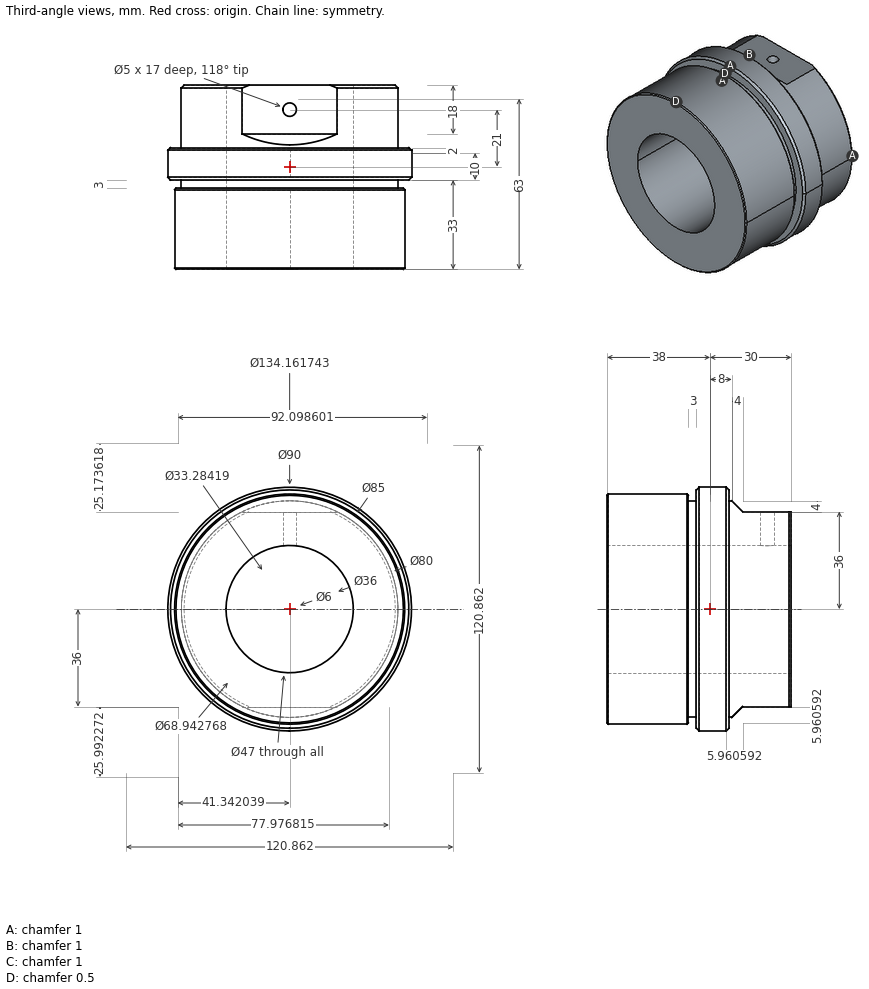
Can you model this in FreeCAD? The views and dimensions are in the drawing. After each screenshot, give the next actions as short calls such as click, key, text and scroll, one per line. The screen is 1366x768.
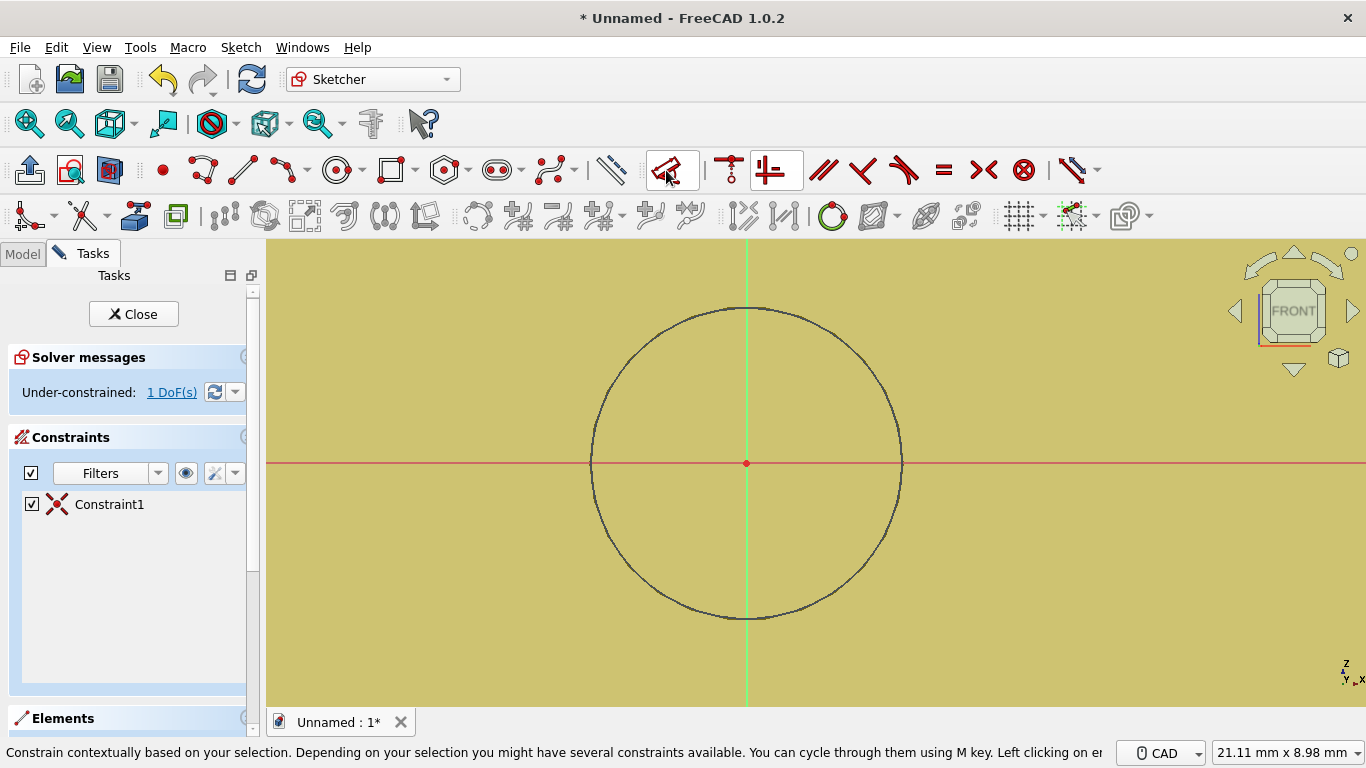
click(856, 353)
click(879, 330)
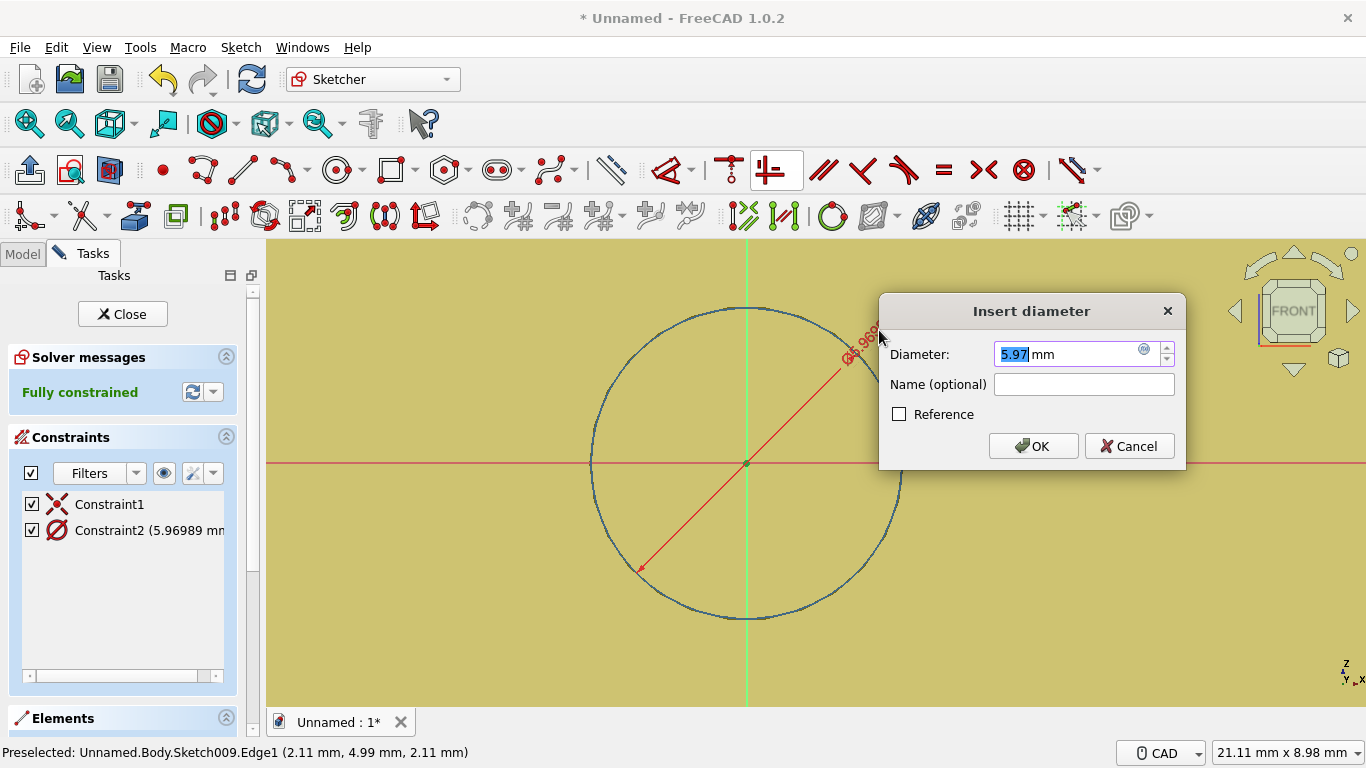
text(6)
key(Return)
key(Escape)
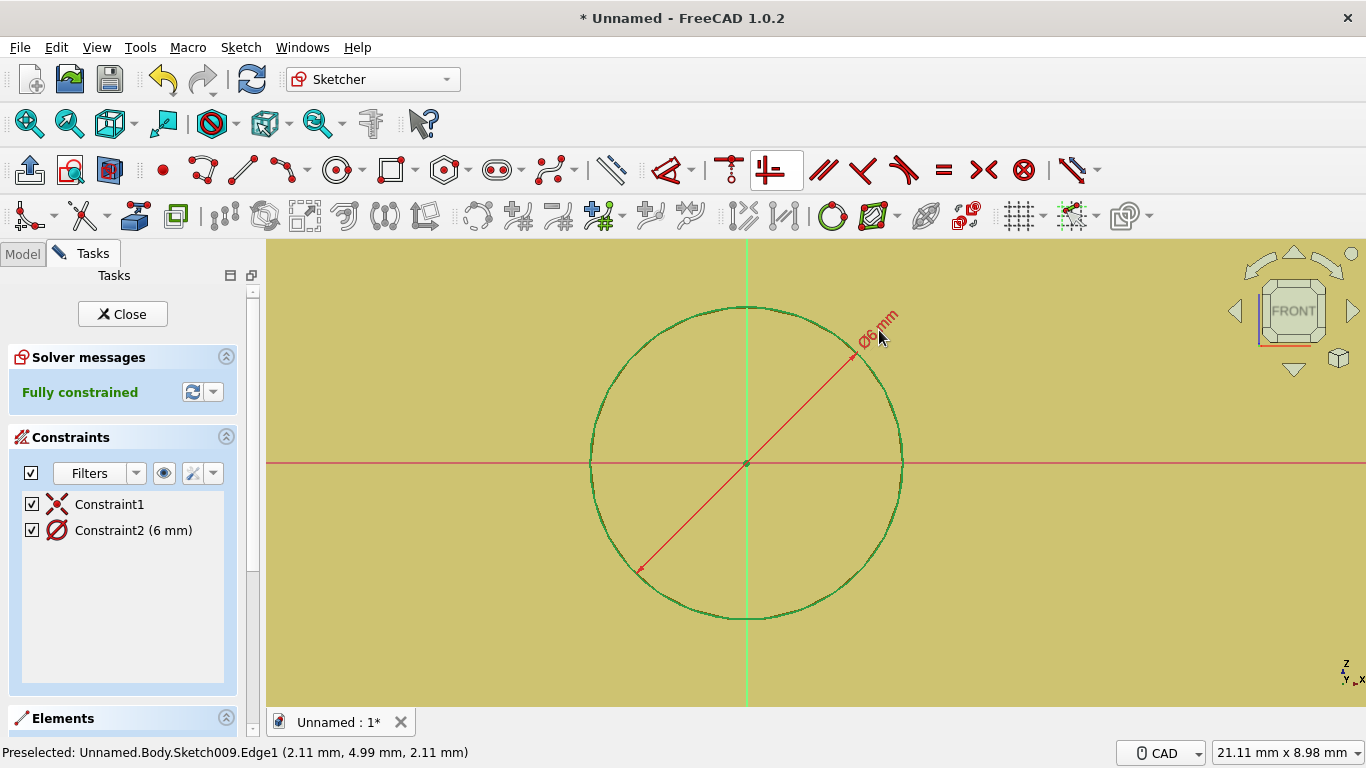
click(123, 314)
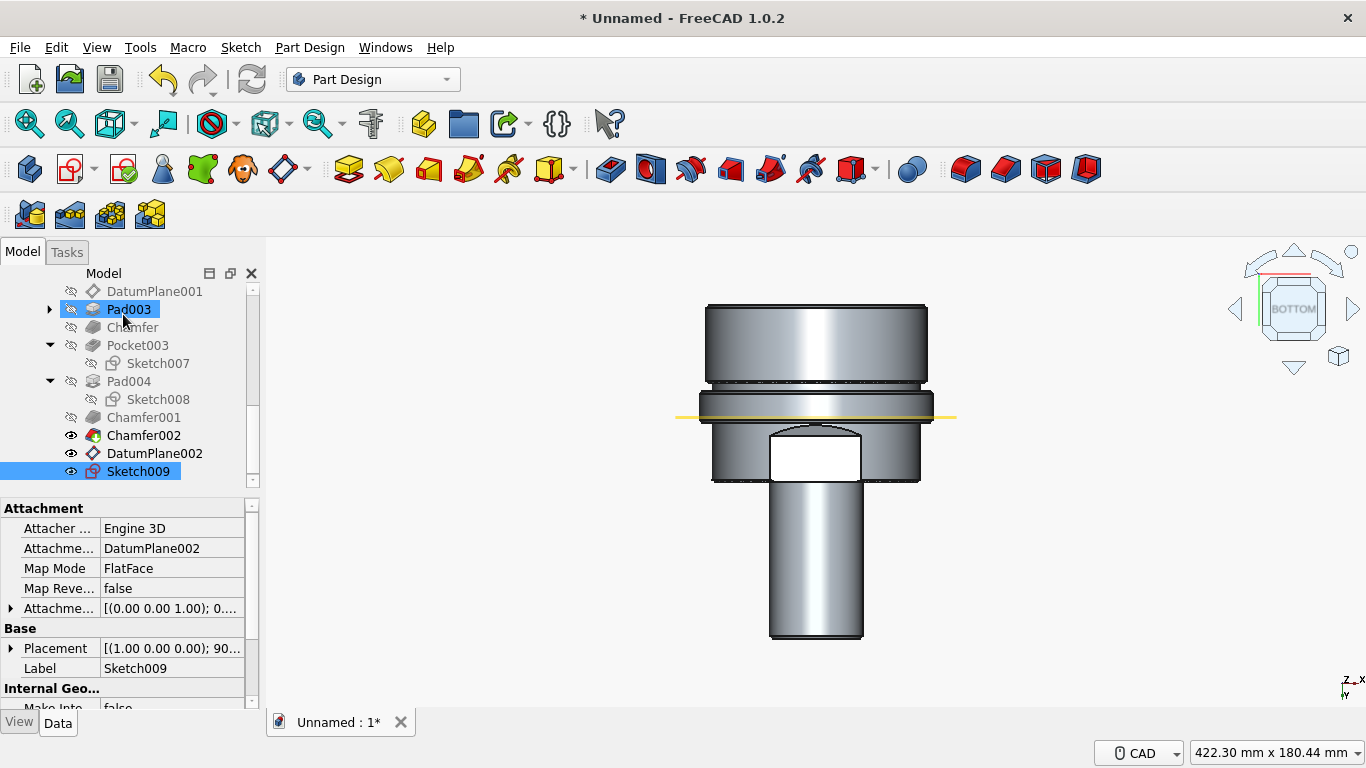
click(612, 170)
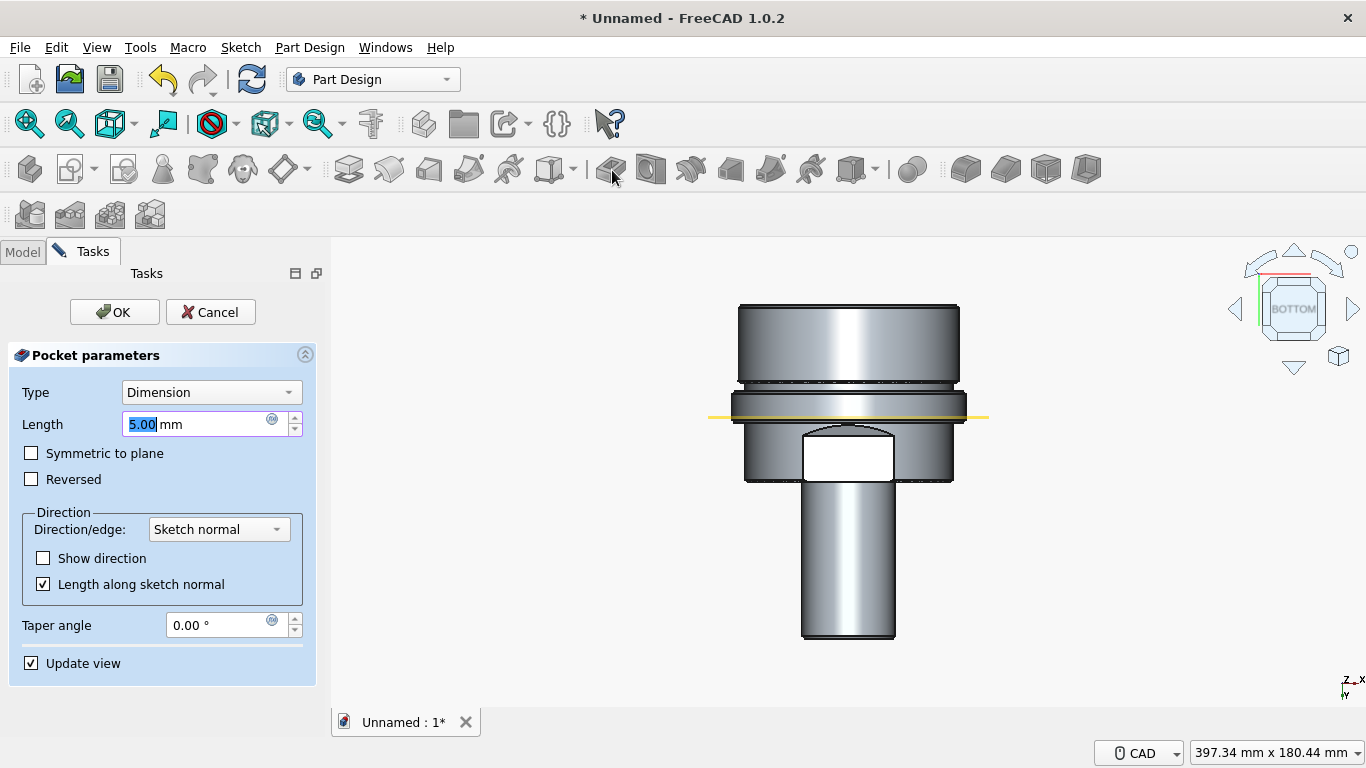
text(2)
key(Tab)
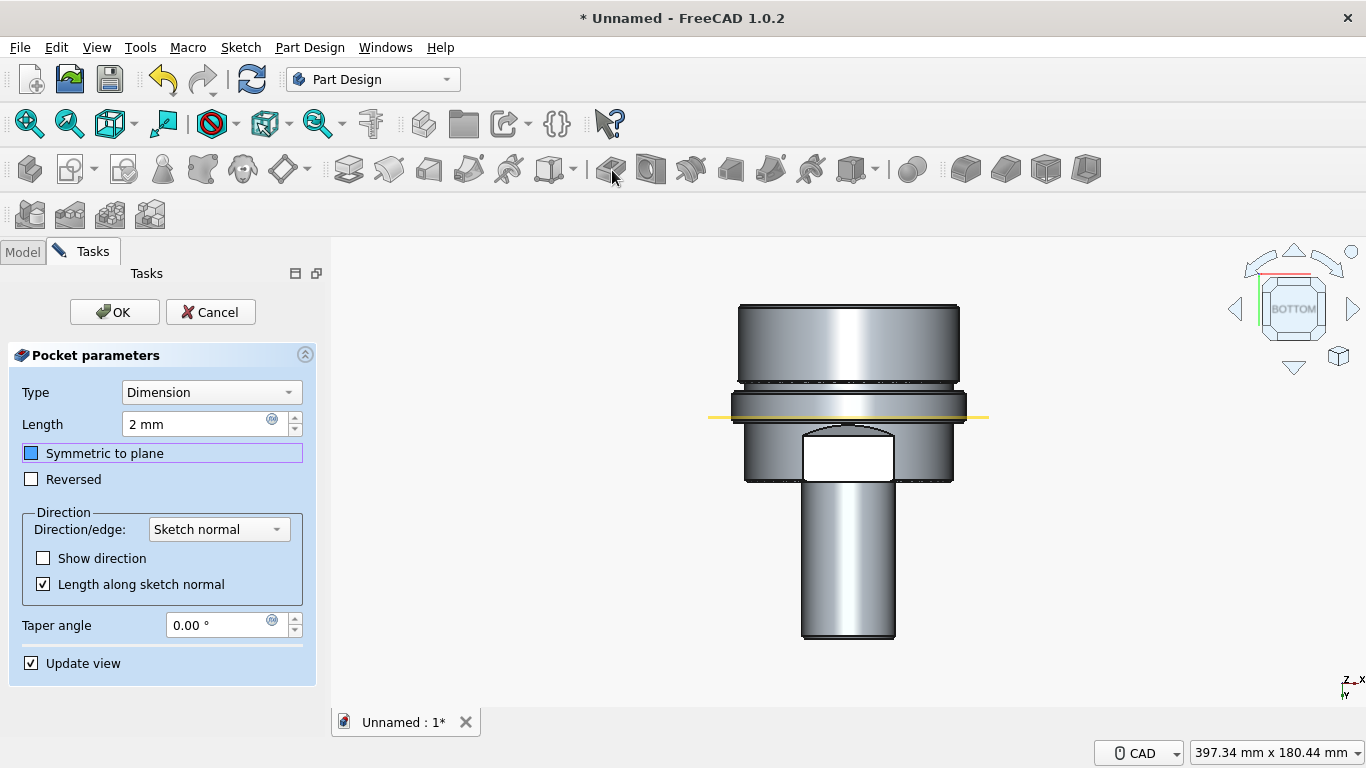
click(115, 312)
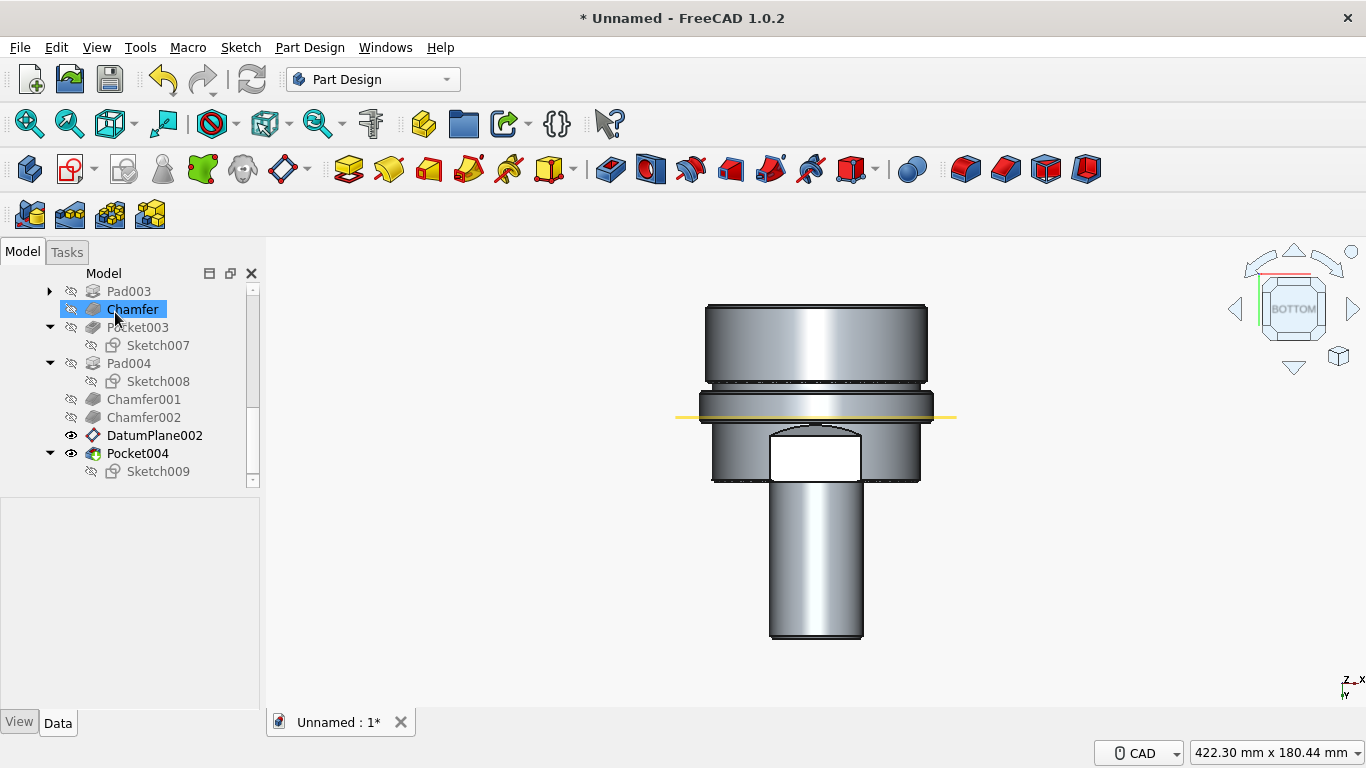
click(116, 435)
key(space)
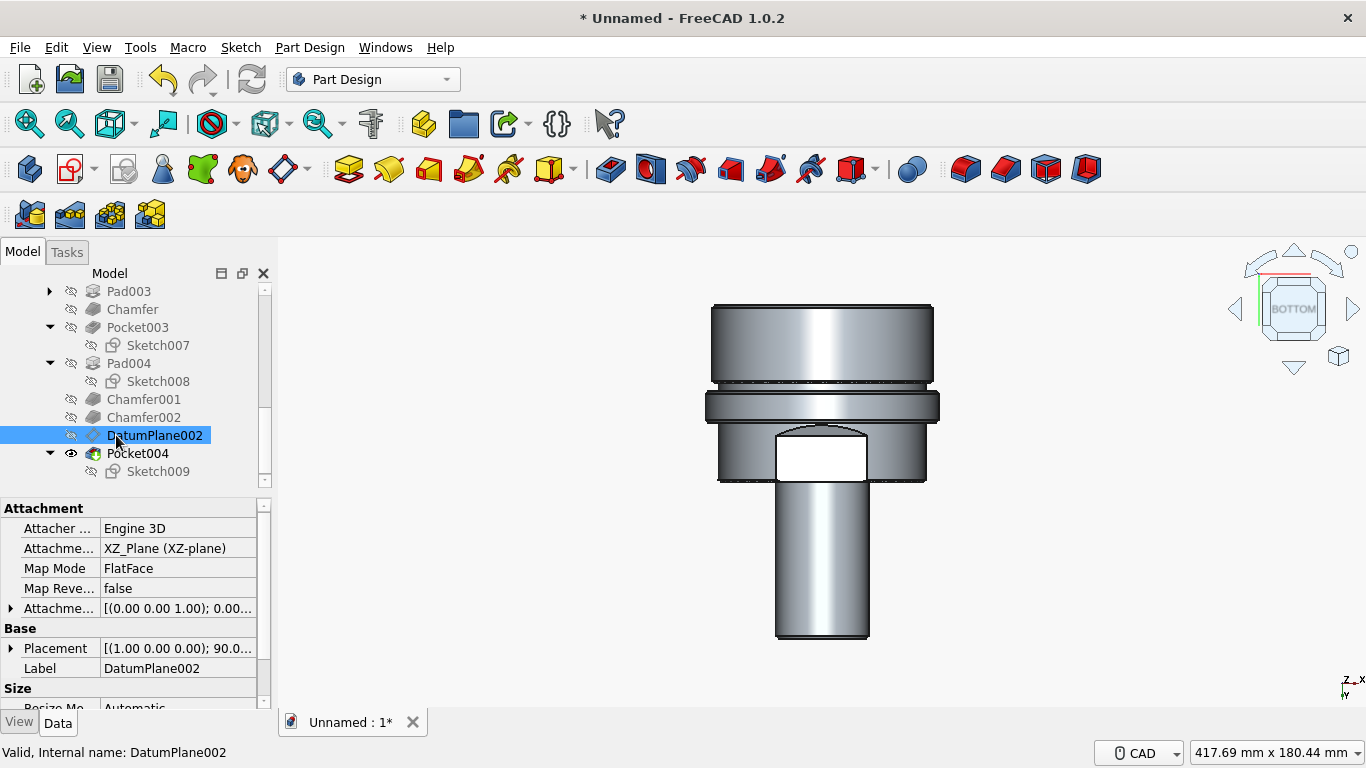
key(4)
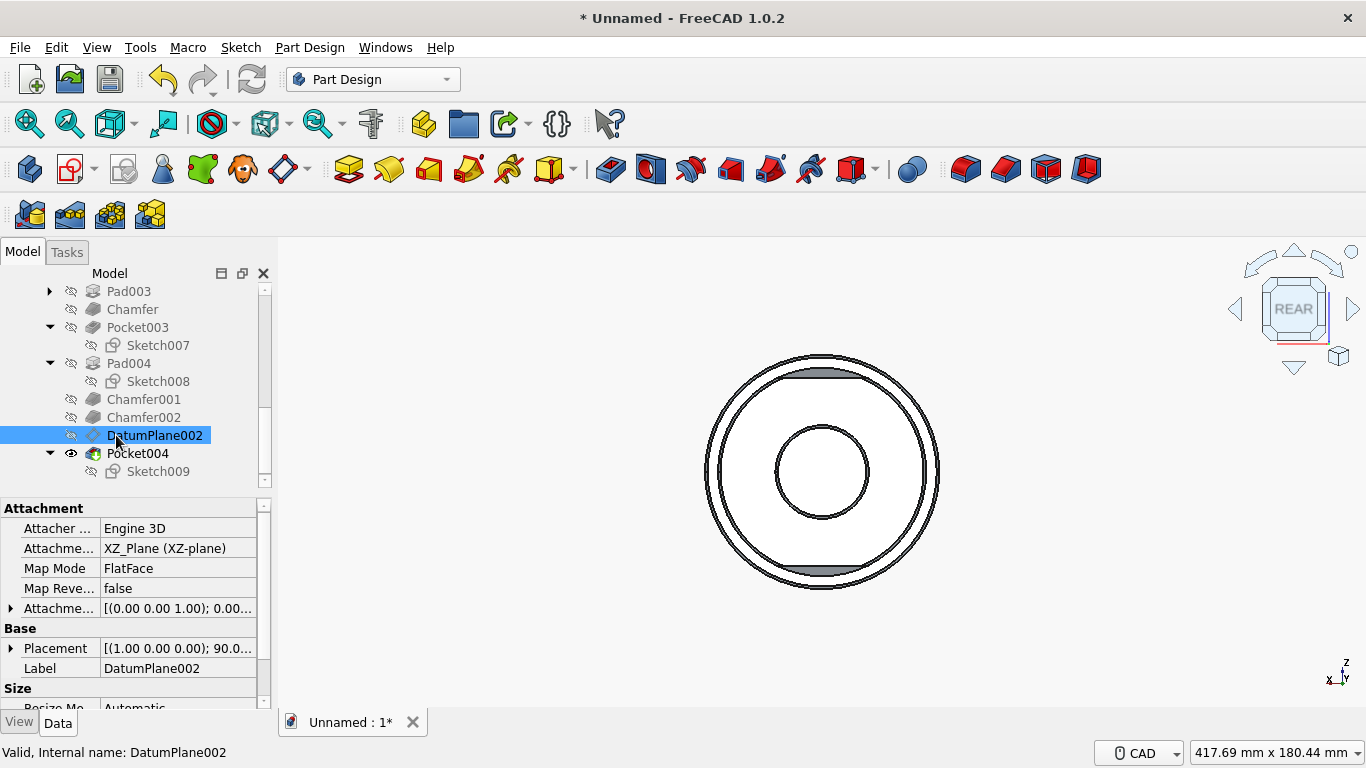
click(764, 525)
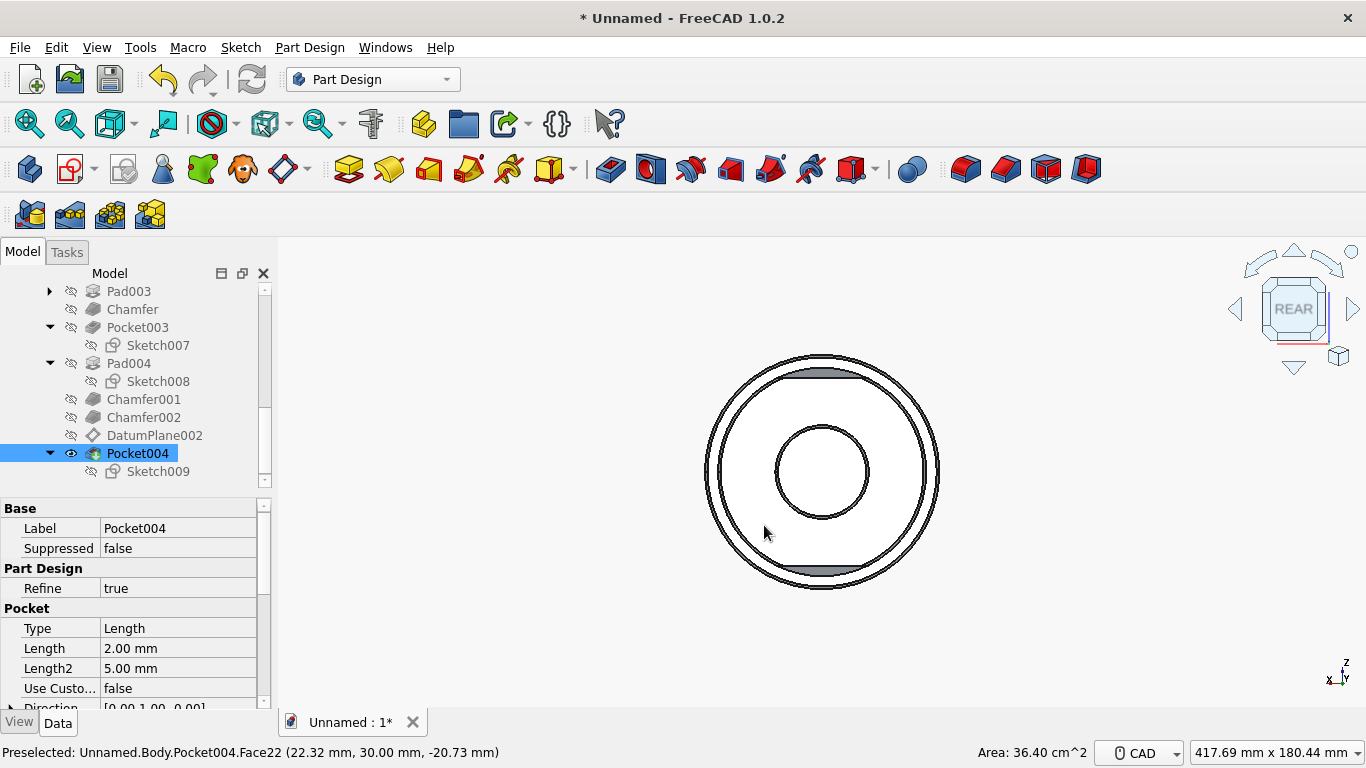
click(70, 170)